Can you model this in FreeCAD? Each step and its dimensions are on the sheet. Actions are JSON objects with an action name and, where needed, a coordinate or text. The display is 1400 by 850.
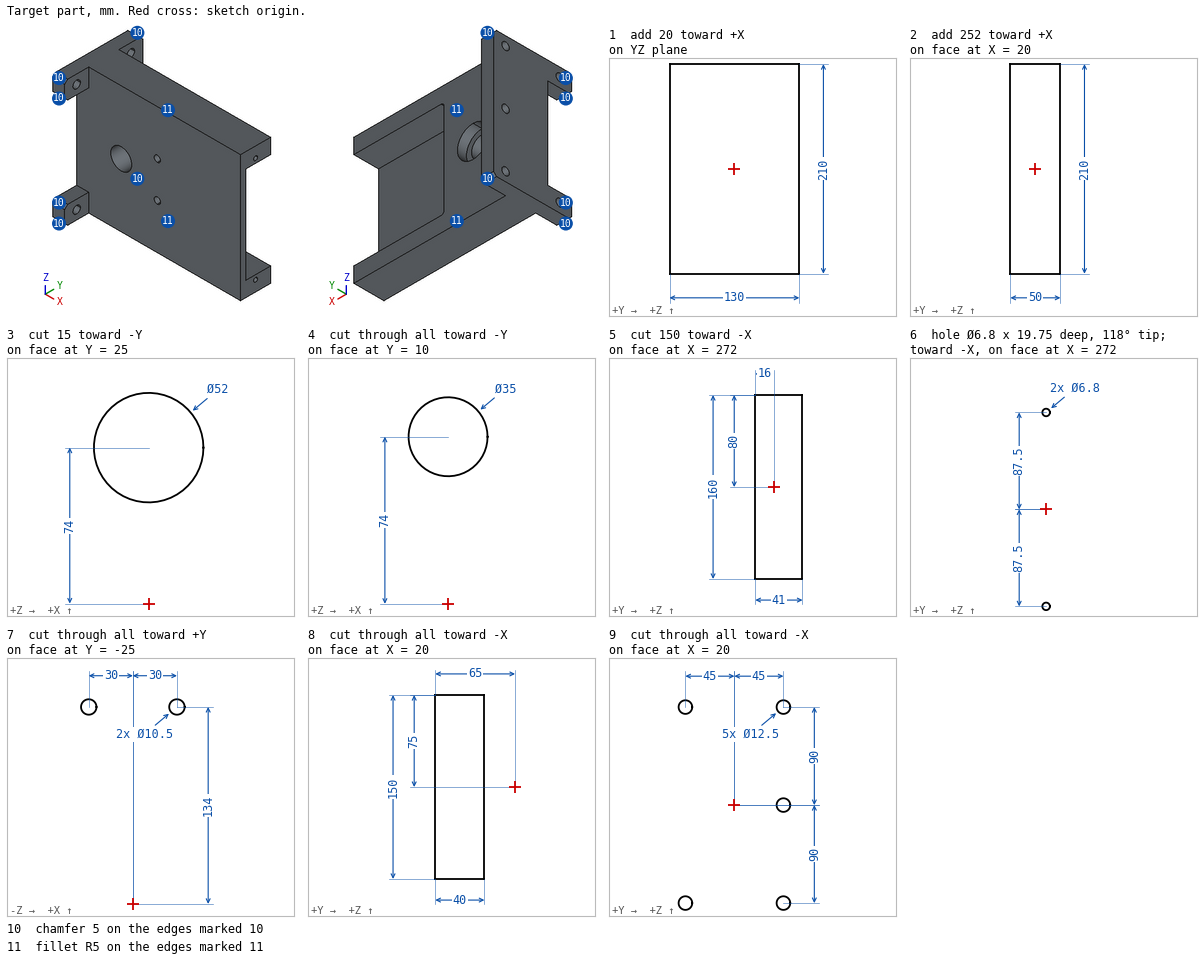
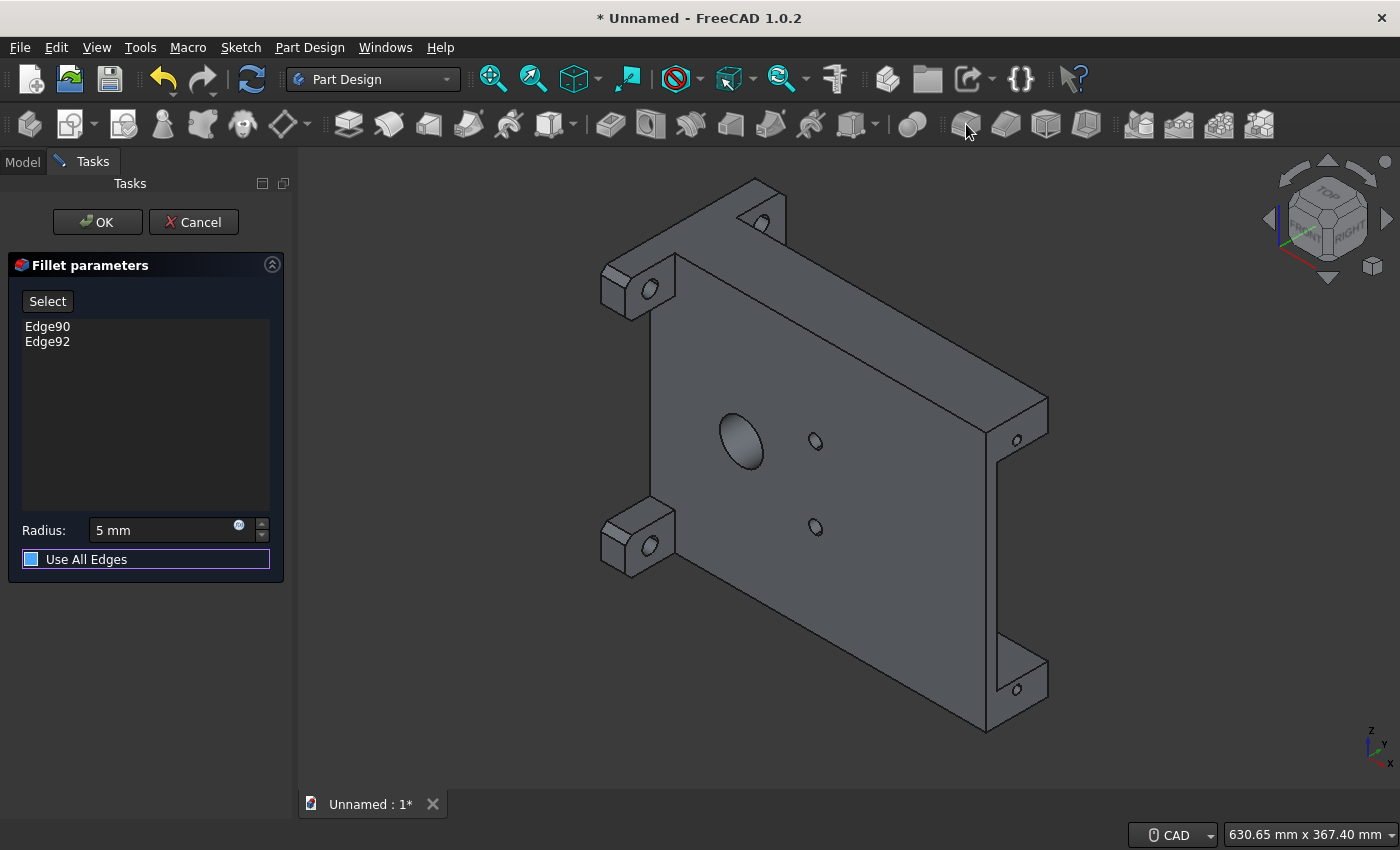
{"action": "left_click", "coordinate": [98, 222]}